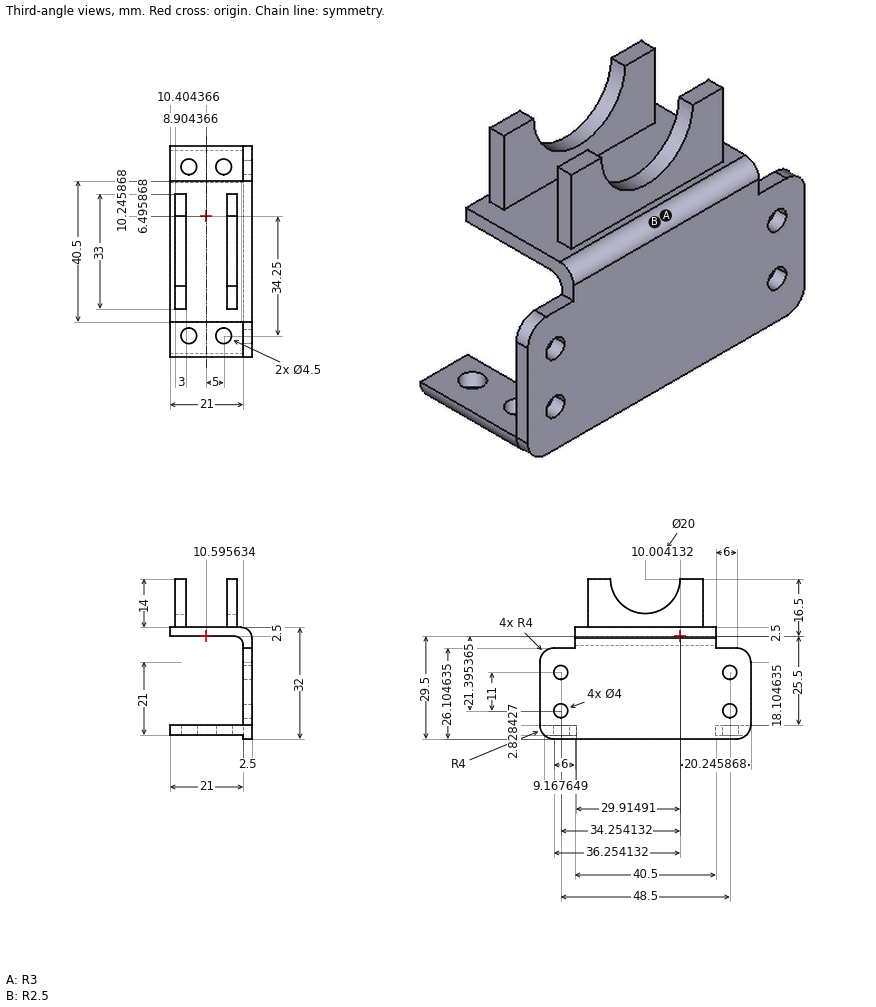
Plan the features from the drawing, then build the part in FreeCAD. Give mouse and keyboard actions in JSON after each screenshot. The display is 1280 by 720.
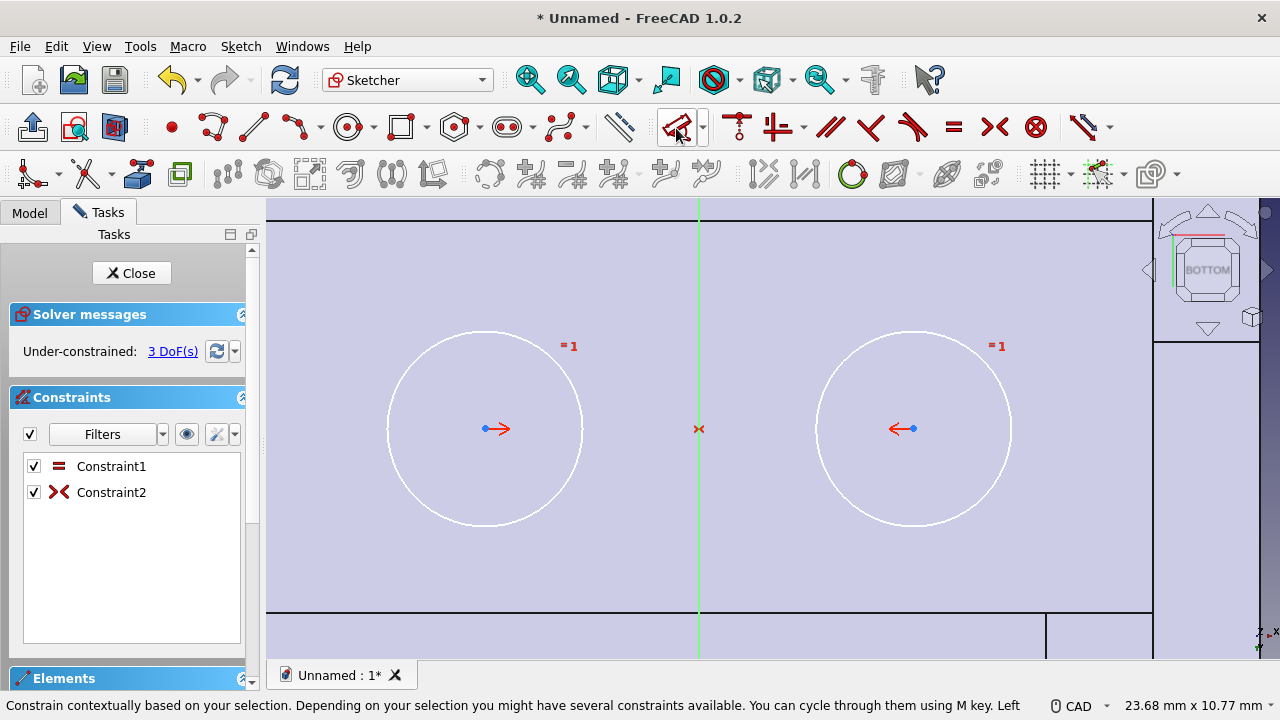
{"action": "left_click", "coordinate": [983, 360]}
{"action": "left_click", "coordinate": [1006, 337]}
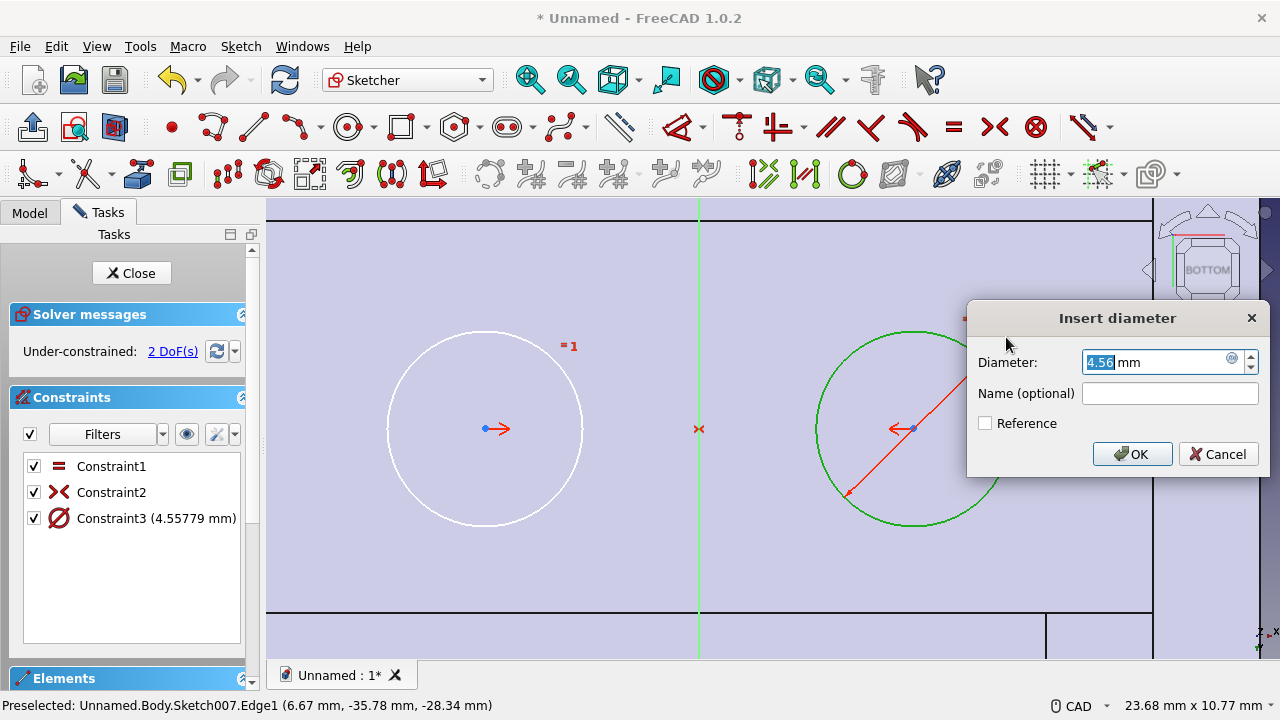
{"action": "type", "text": "4.5"}
{"action": "key", "text": "Return"}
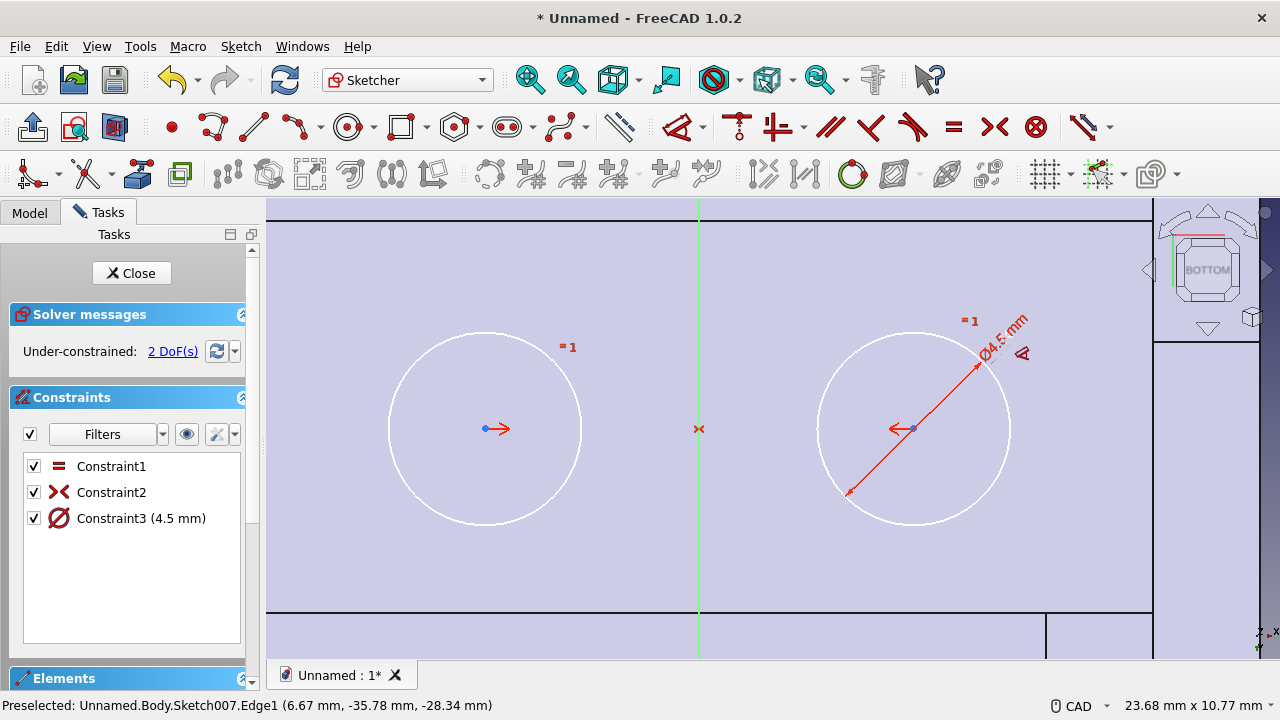
{"action": "left_click", "coordinate": [914, 429]}
{"action": "left_click", "coordinate": [807, 395]}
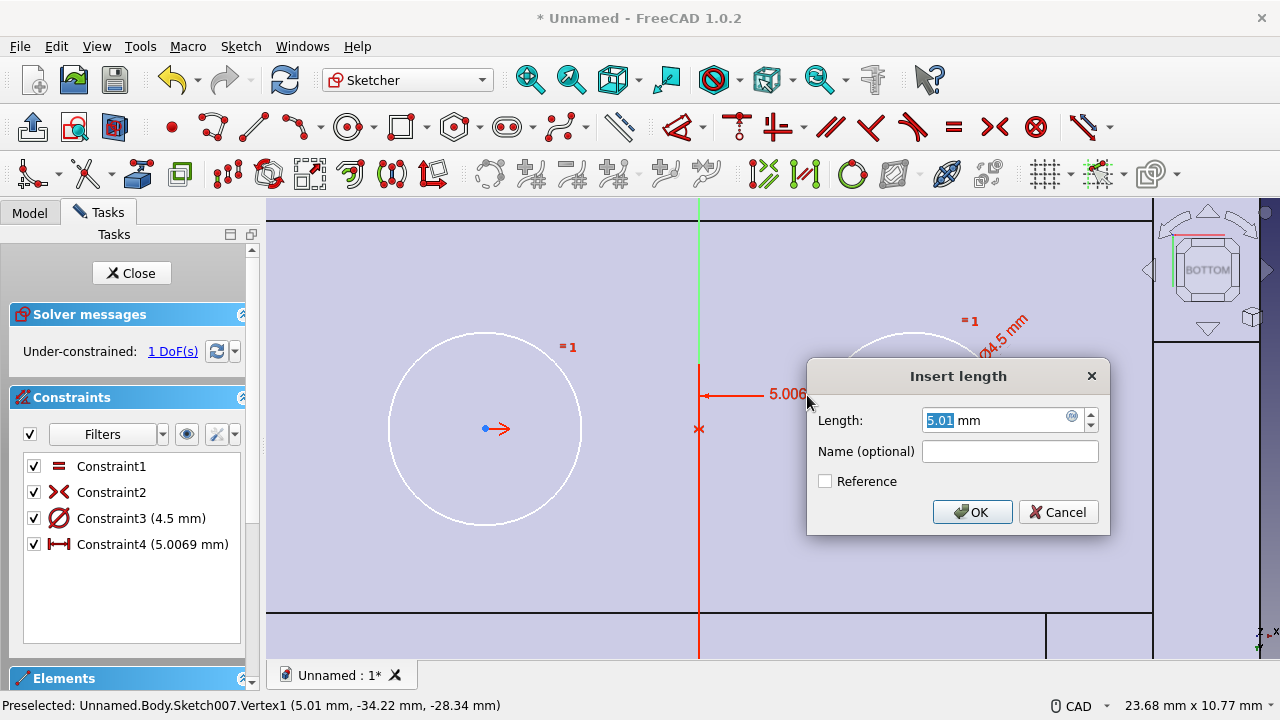
{"action": "type", "text": "5"}
{"action": "key", "text": "Return"}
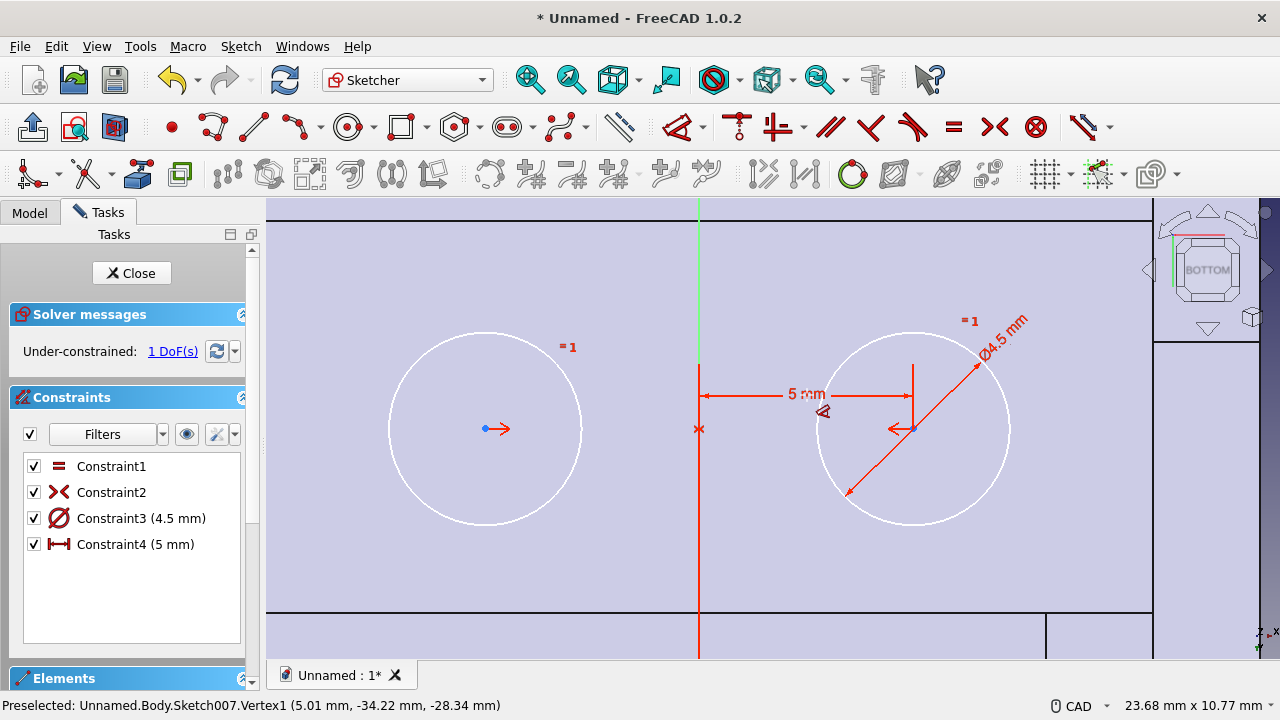
{"action": "left_click", "coordinate": [913, 429]}
{"action": "left_click", "coordinate": [947, 484]}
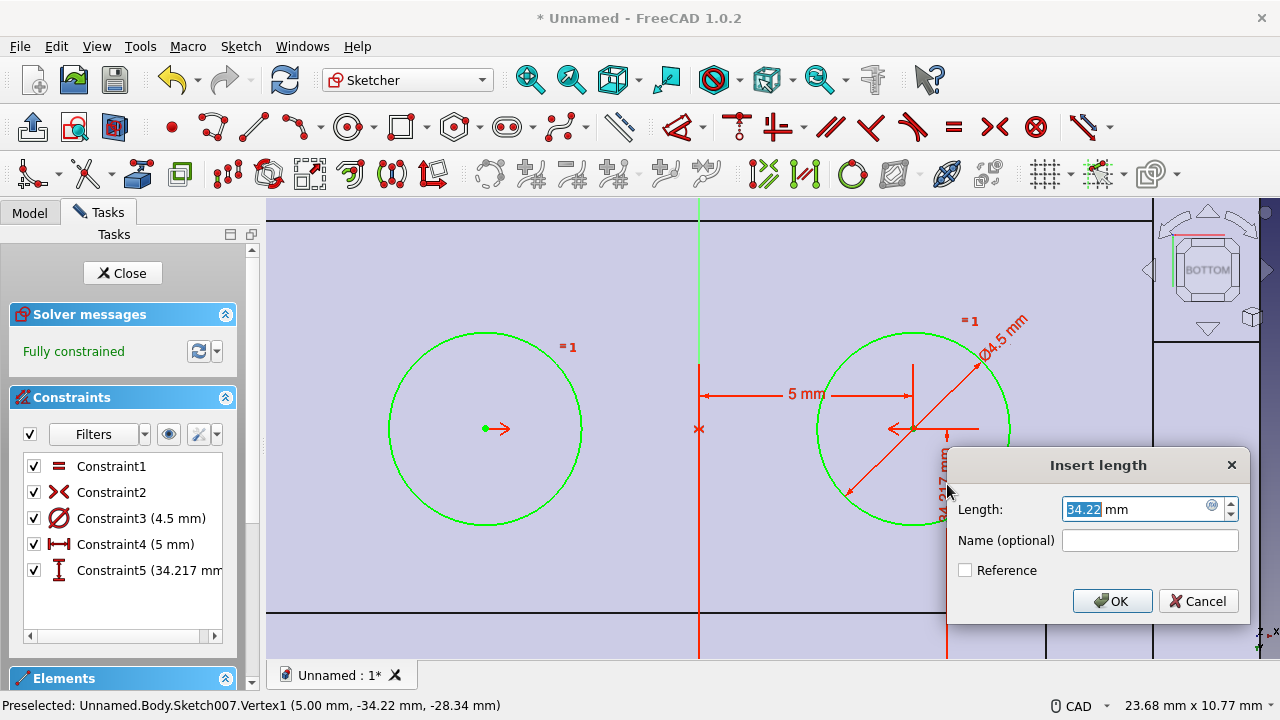
{"action": "type", "text": "34.25"}
{"action": "key", "text": "Return"}
{"action": "key", "text": "Escape"}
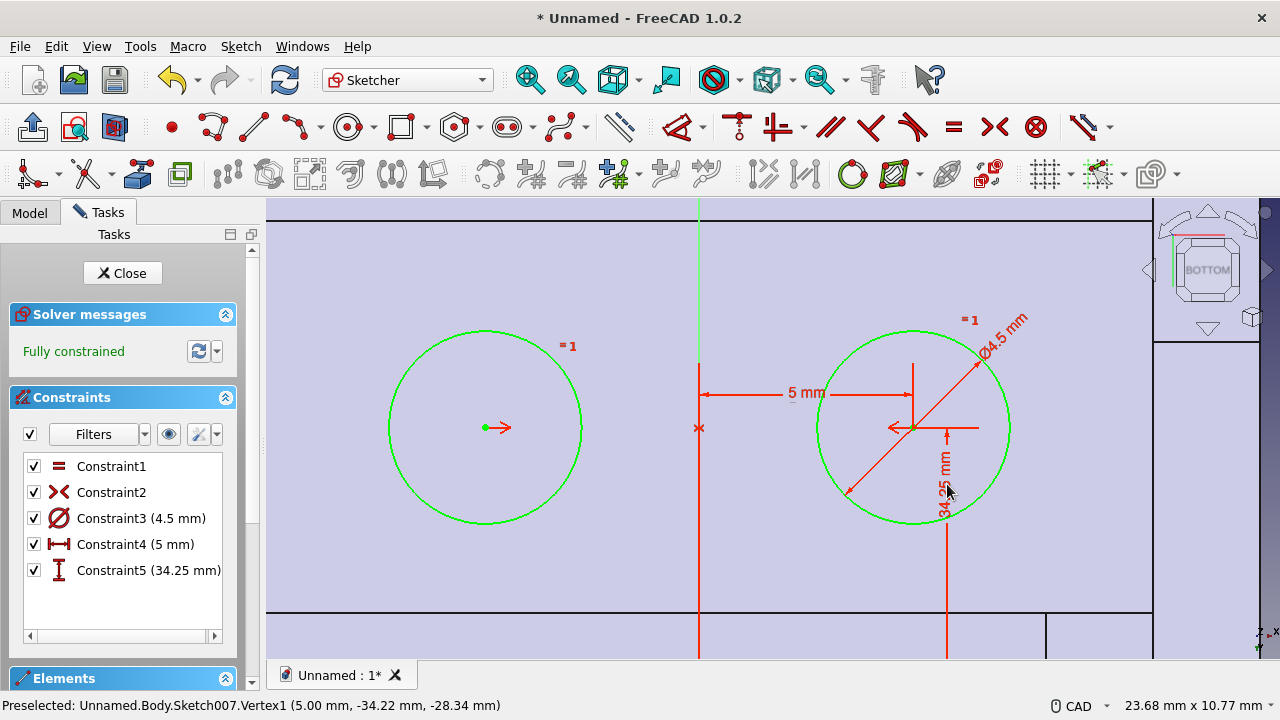
{"action": "left_click", "coordinate": [123, 273]}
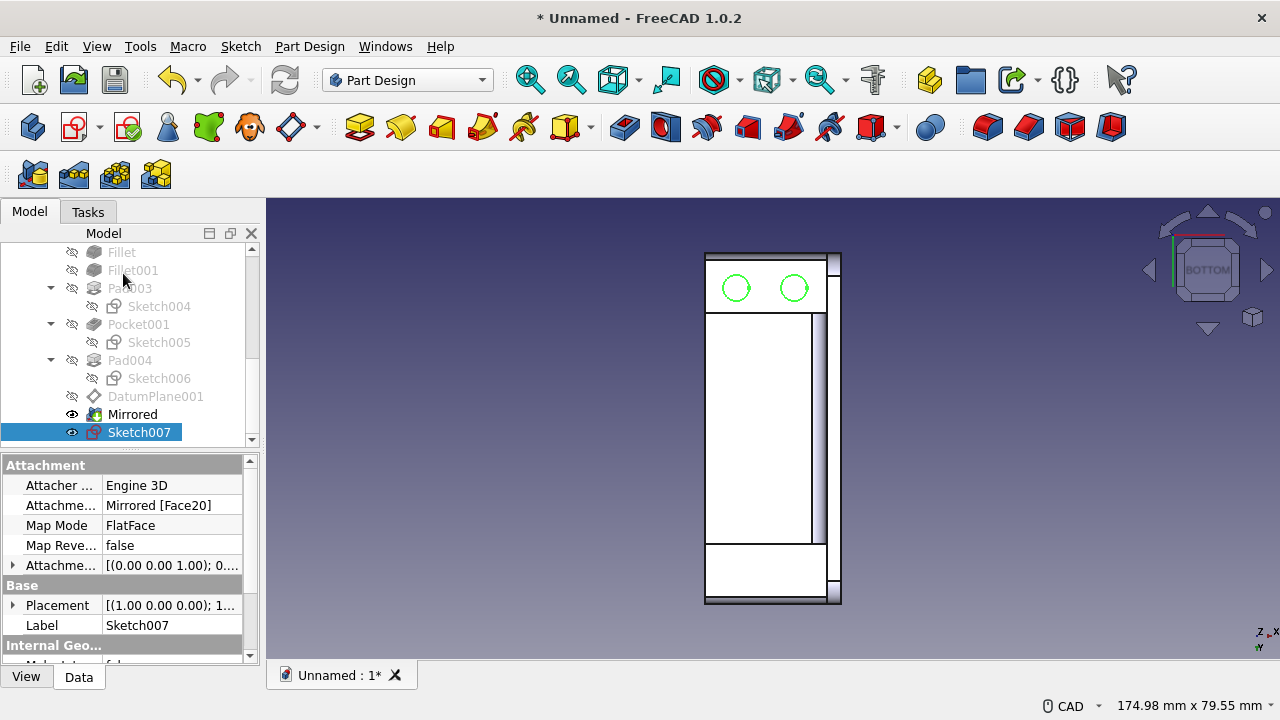
{"action": "left_click", "coordinate": [625, 128]}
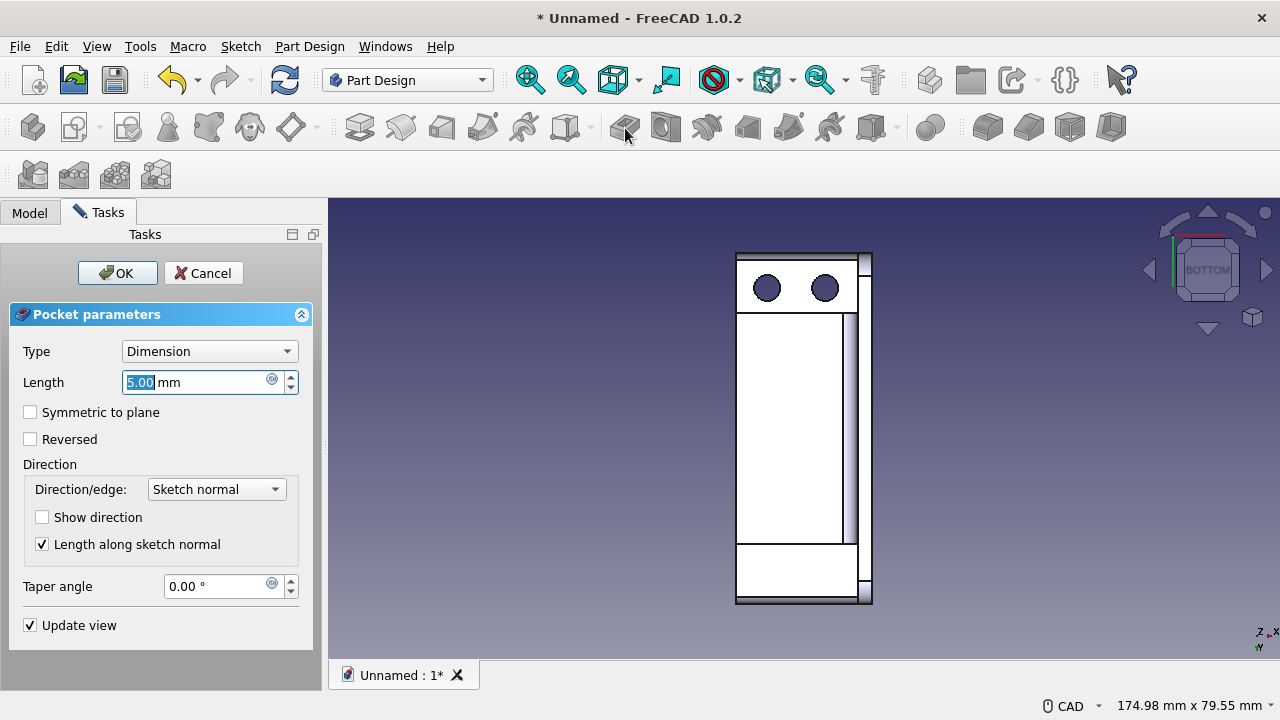
{"action": "type", "text": "21"}
{"action": "key", "text": "Tab"}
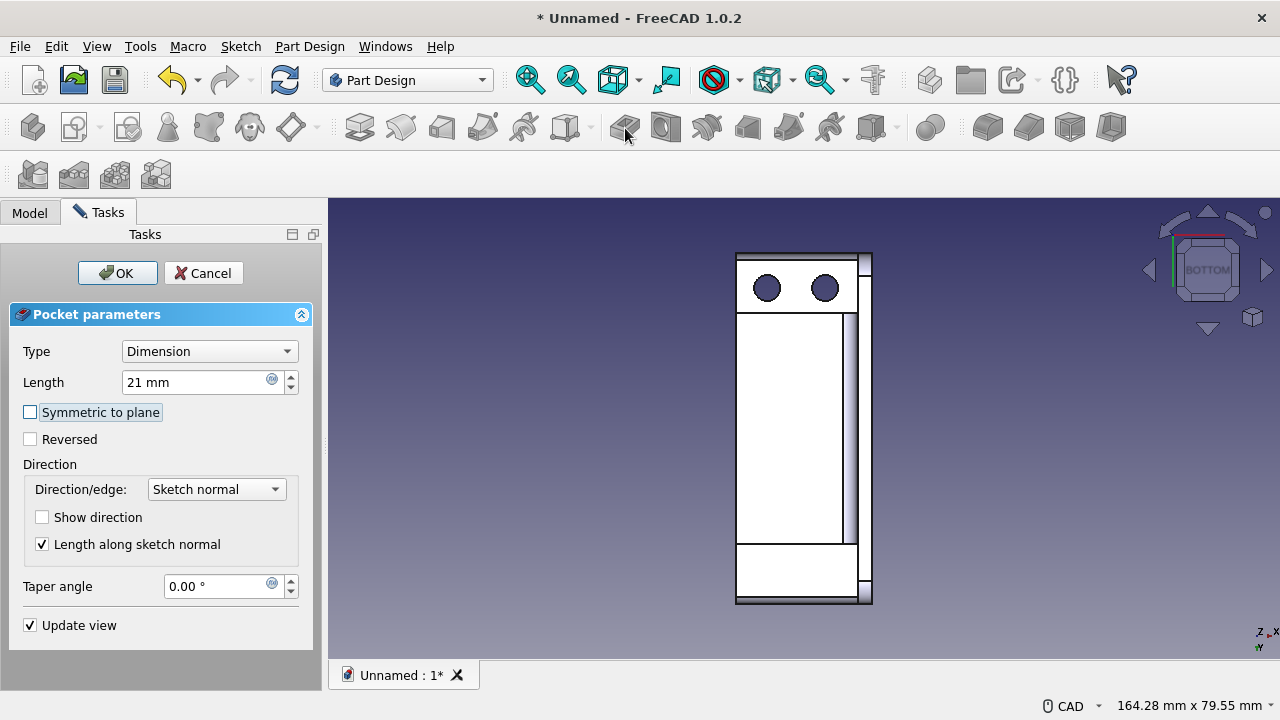
{"action": "left_click", "coordinate": [118, 273]}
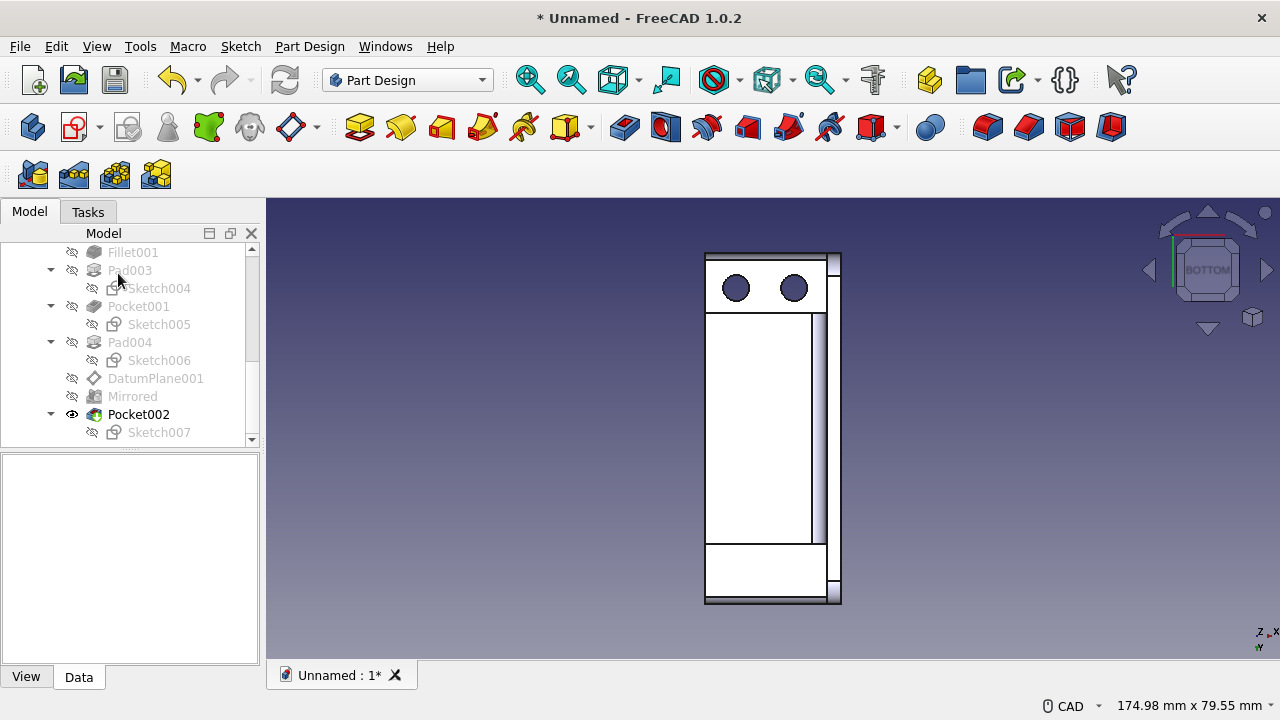
{"action": "scroll", "coordinate": [141, 338], "scroll_direction": "down", "scroll_amount": 3}